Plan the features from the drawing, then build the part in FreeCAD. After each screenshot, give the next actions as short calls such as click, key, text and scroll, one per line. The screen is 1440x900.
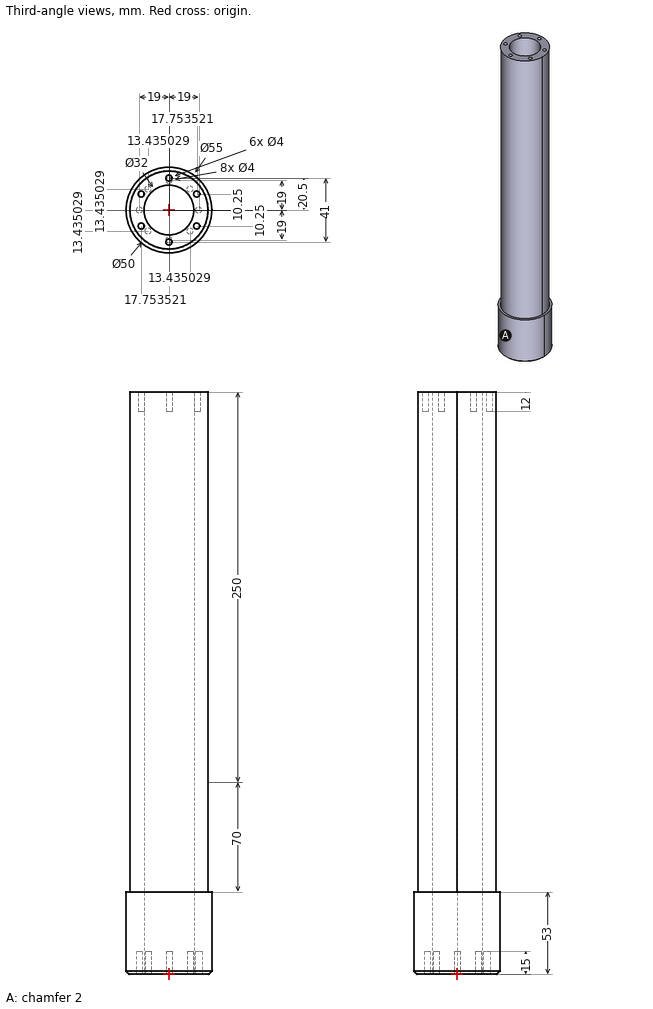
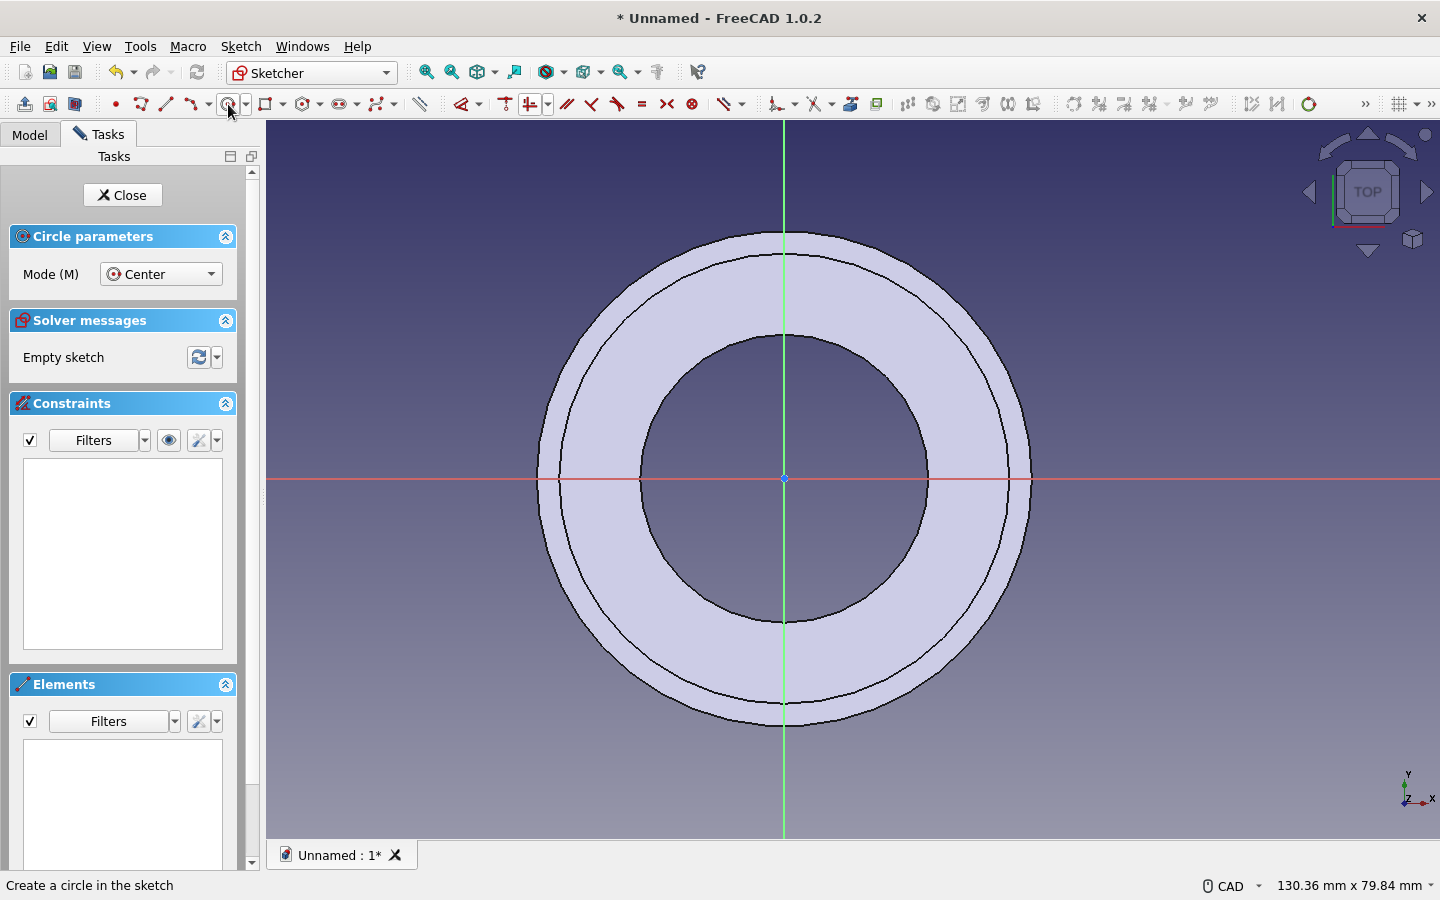
click(784, 479)
move(943, 319)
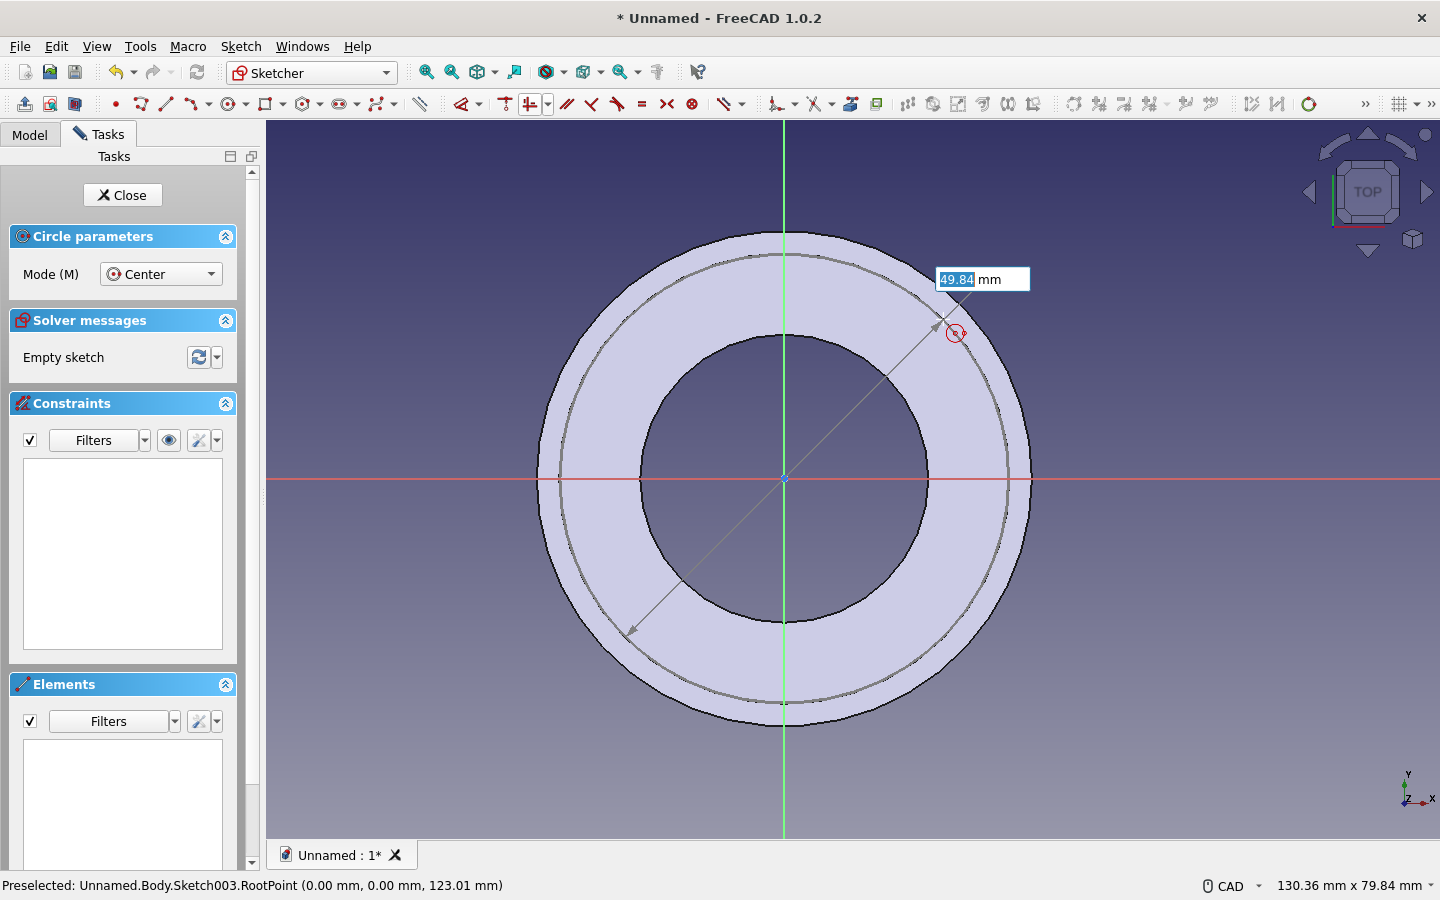
text(50)
key(Return)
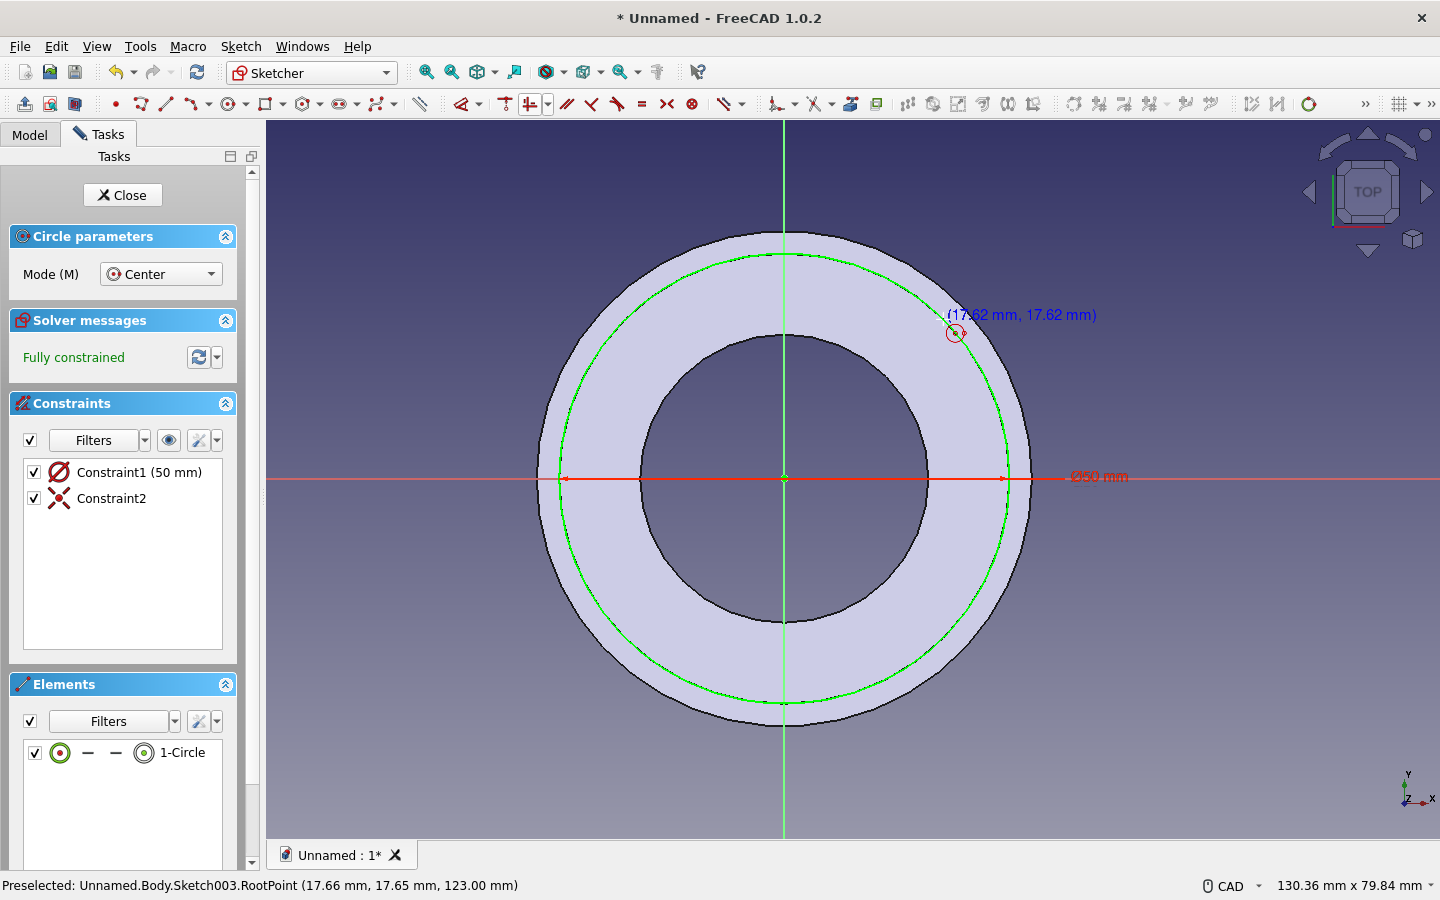
click(784, 479)
move(886, 377)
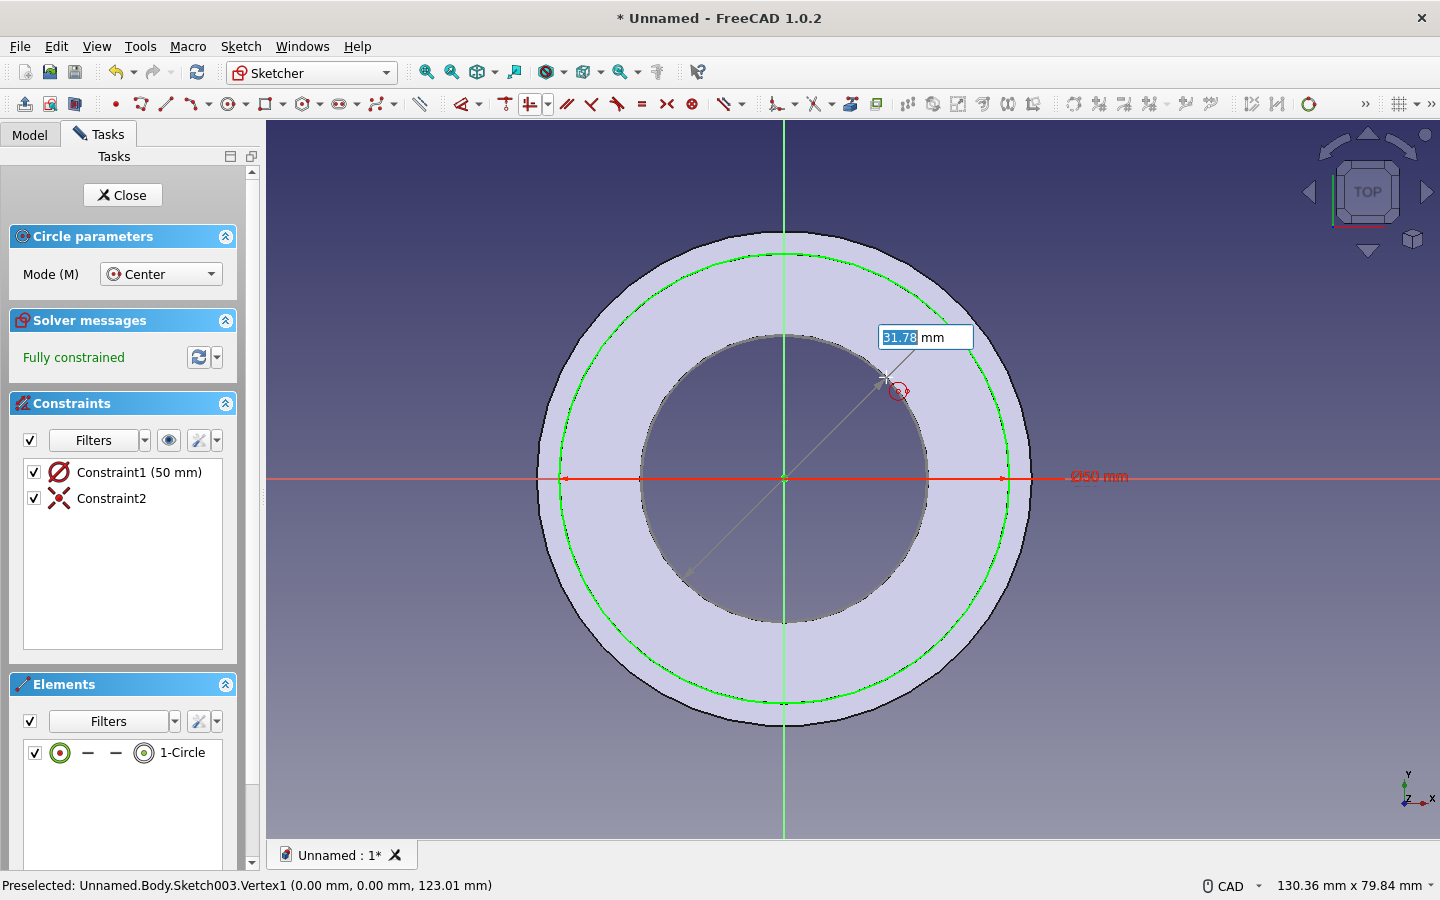
text(32)
key(Return)
key(Escape)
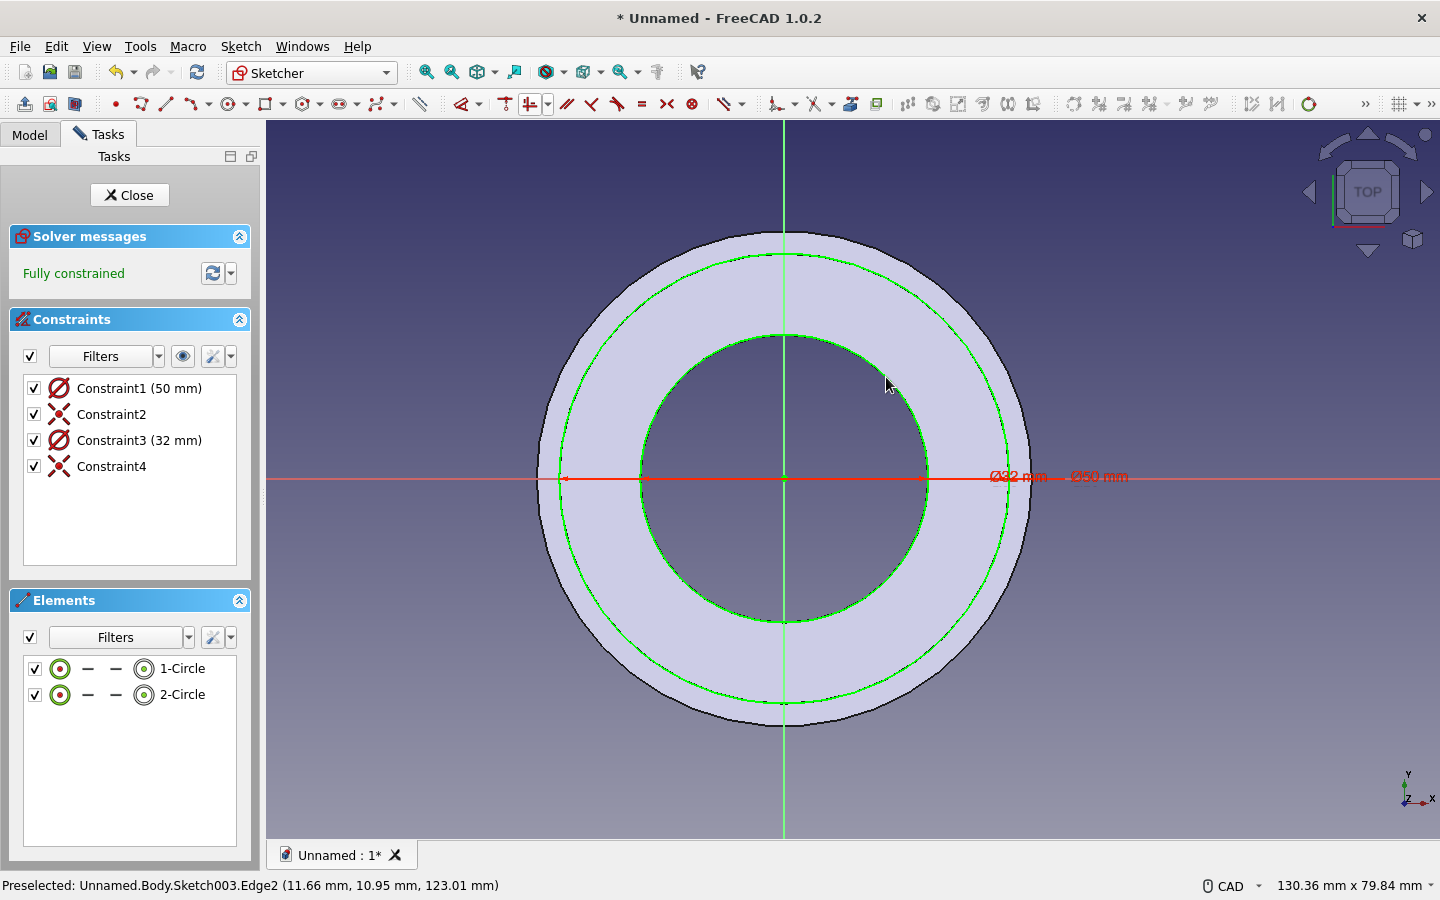
click(130, 195)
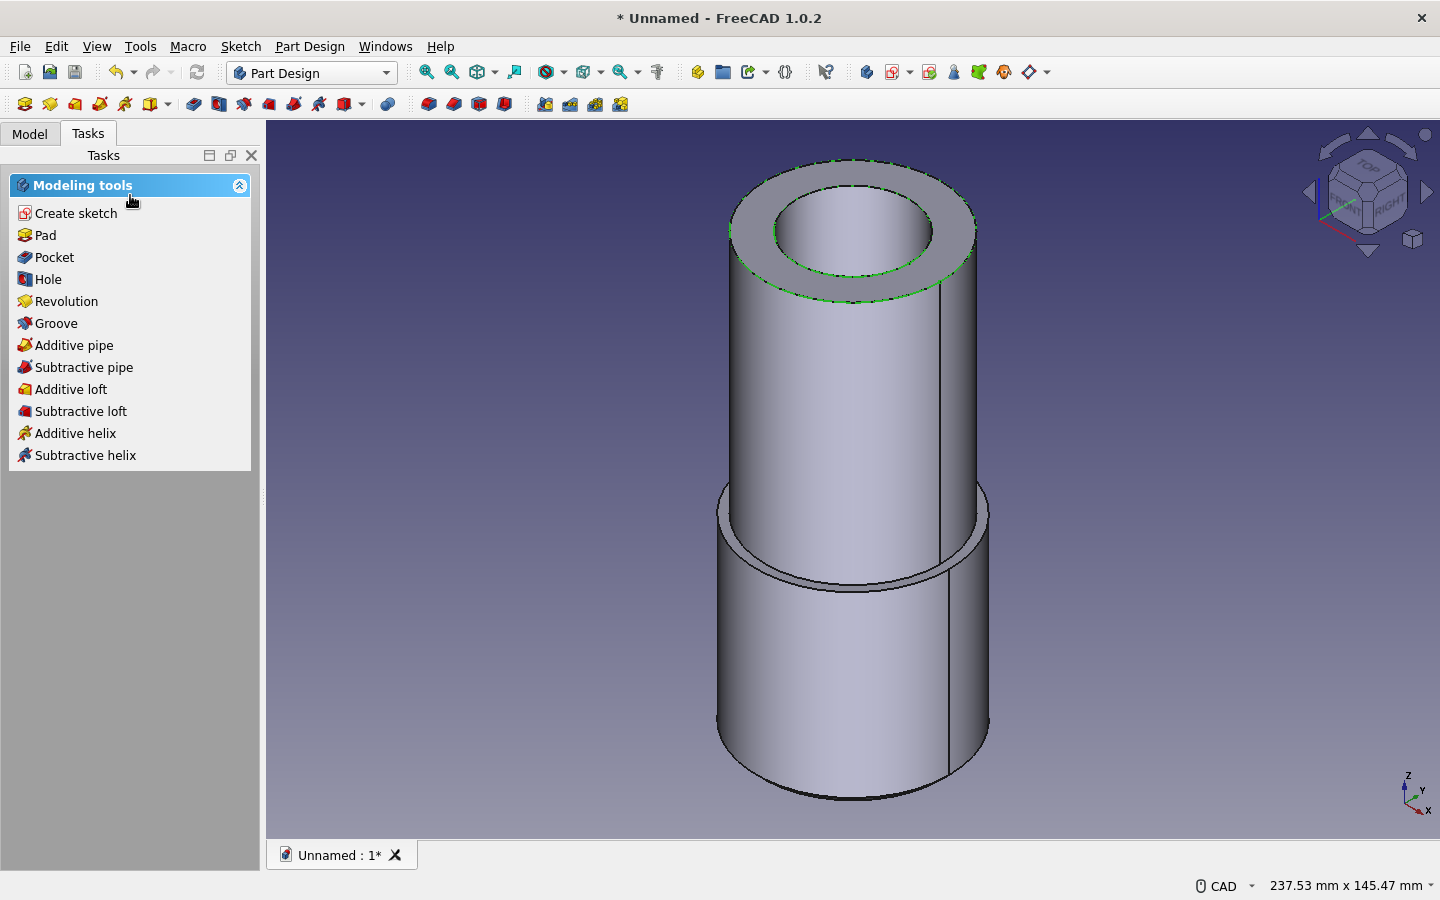
click(25, 104)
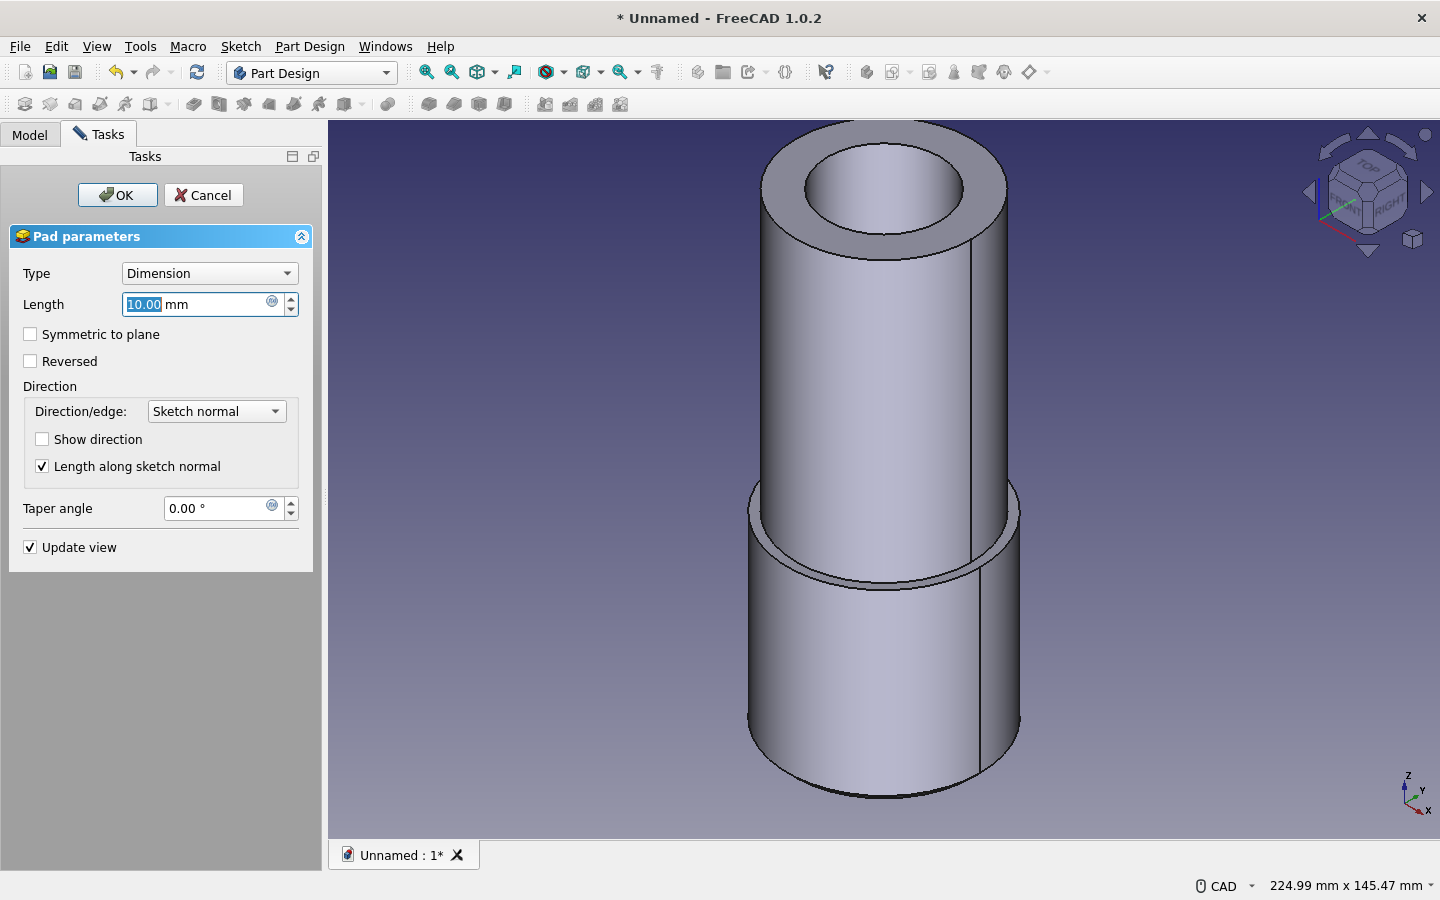
text(250)
key(Tab)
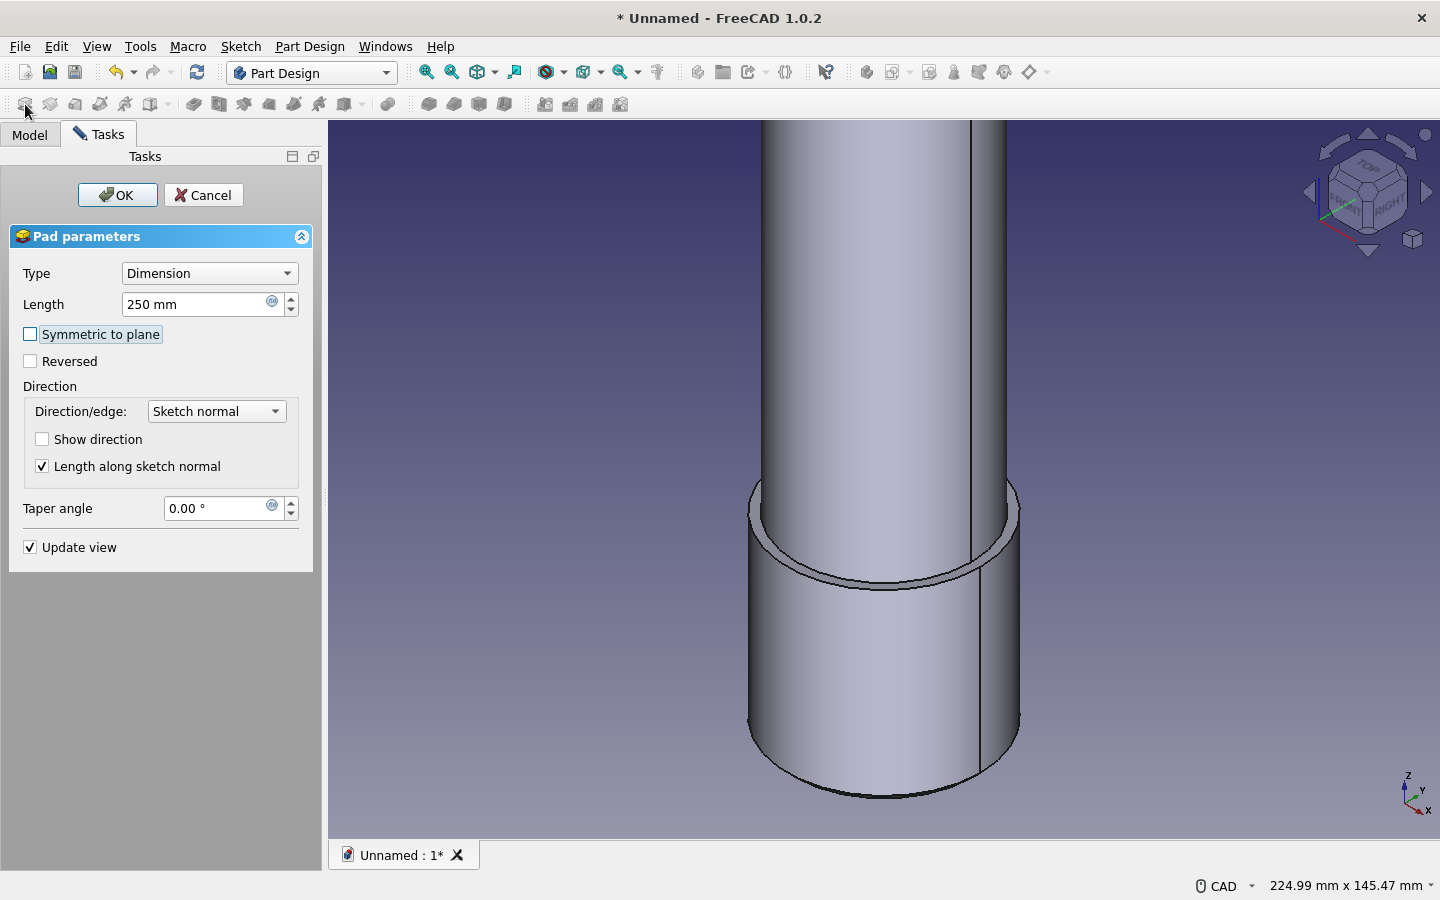
click(118, 195)